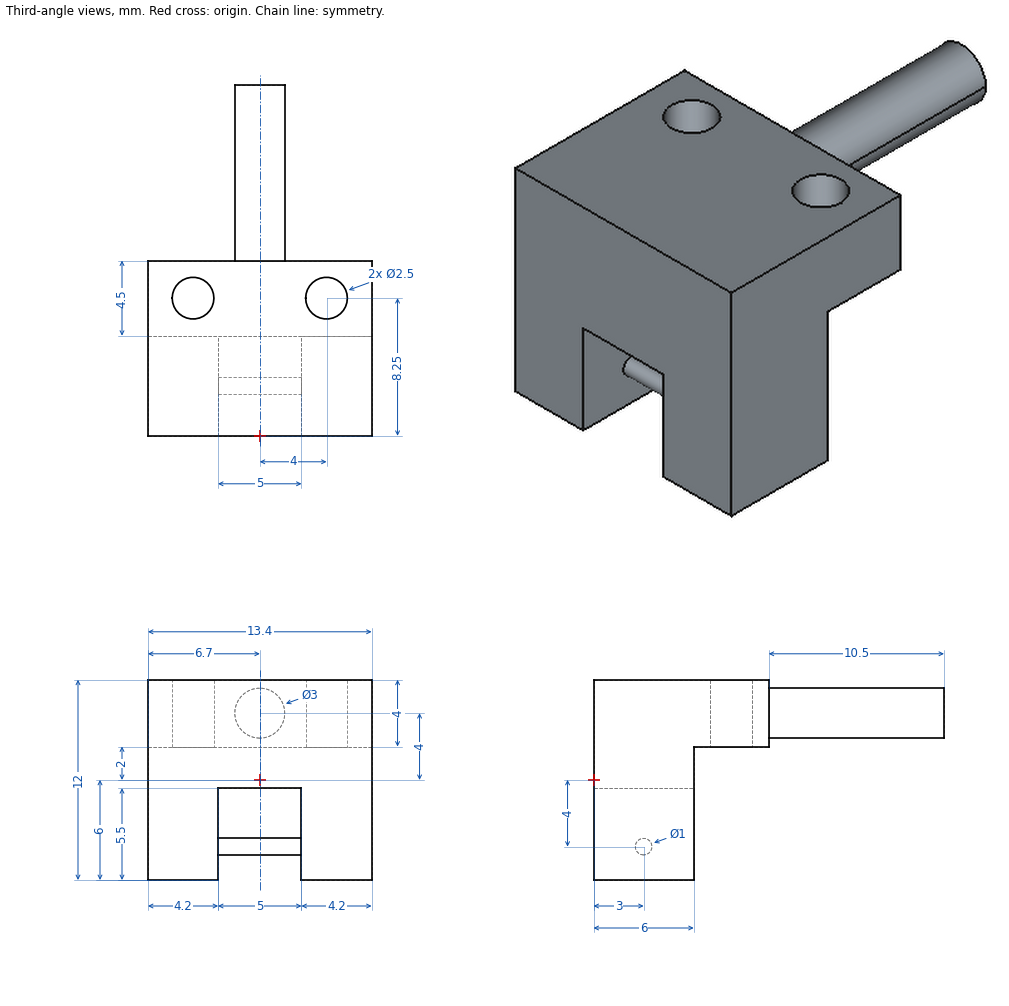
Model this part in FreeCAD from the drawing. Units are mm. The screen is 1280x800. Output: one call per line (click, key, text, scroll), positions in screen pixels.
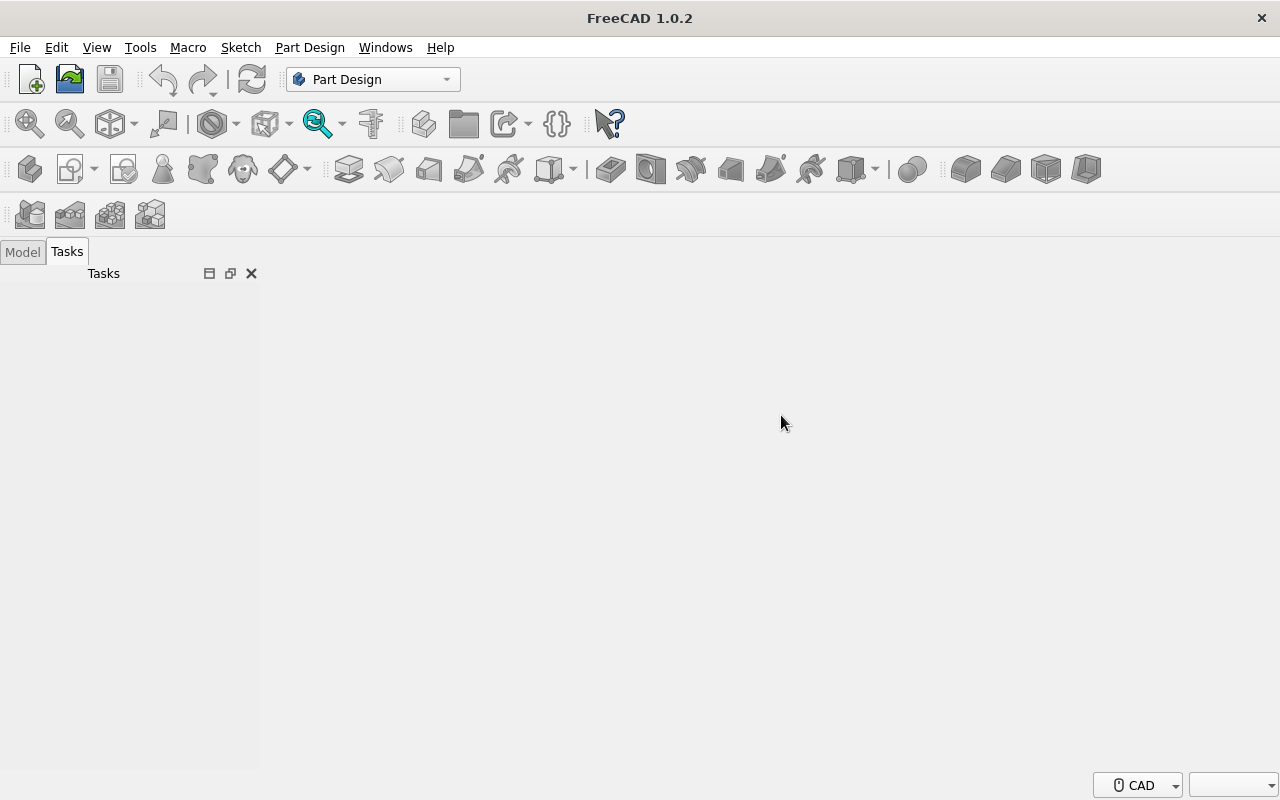
click(30, 80)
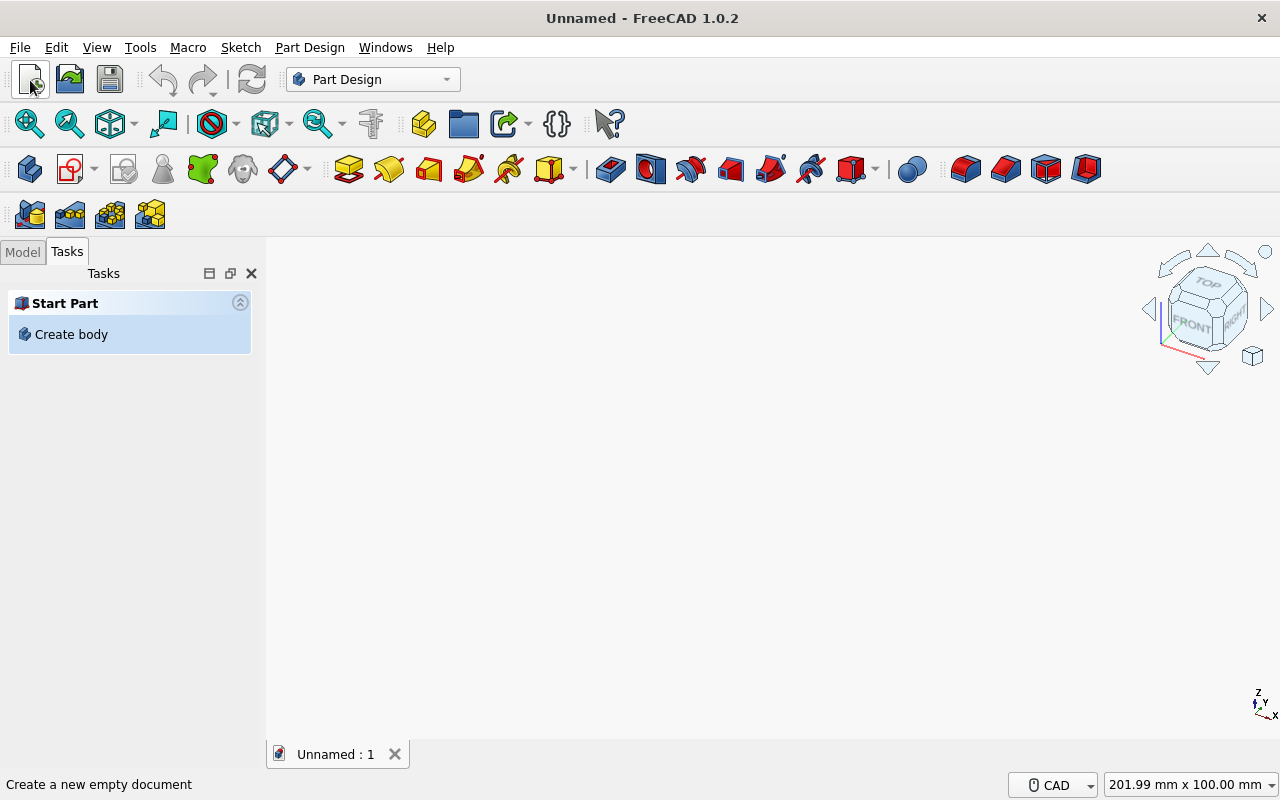
click(70, 170)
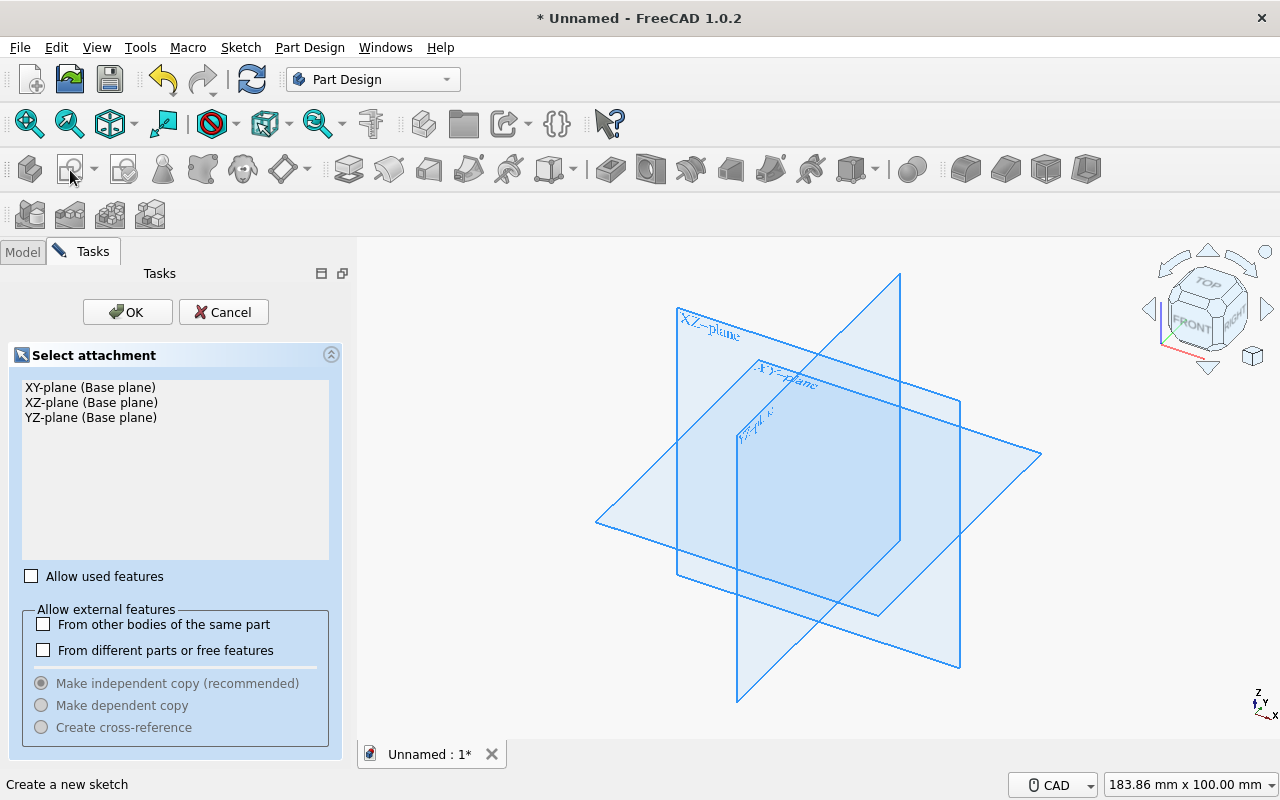
click(82, 402)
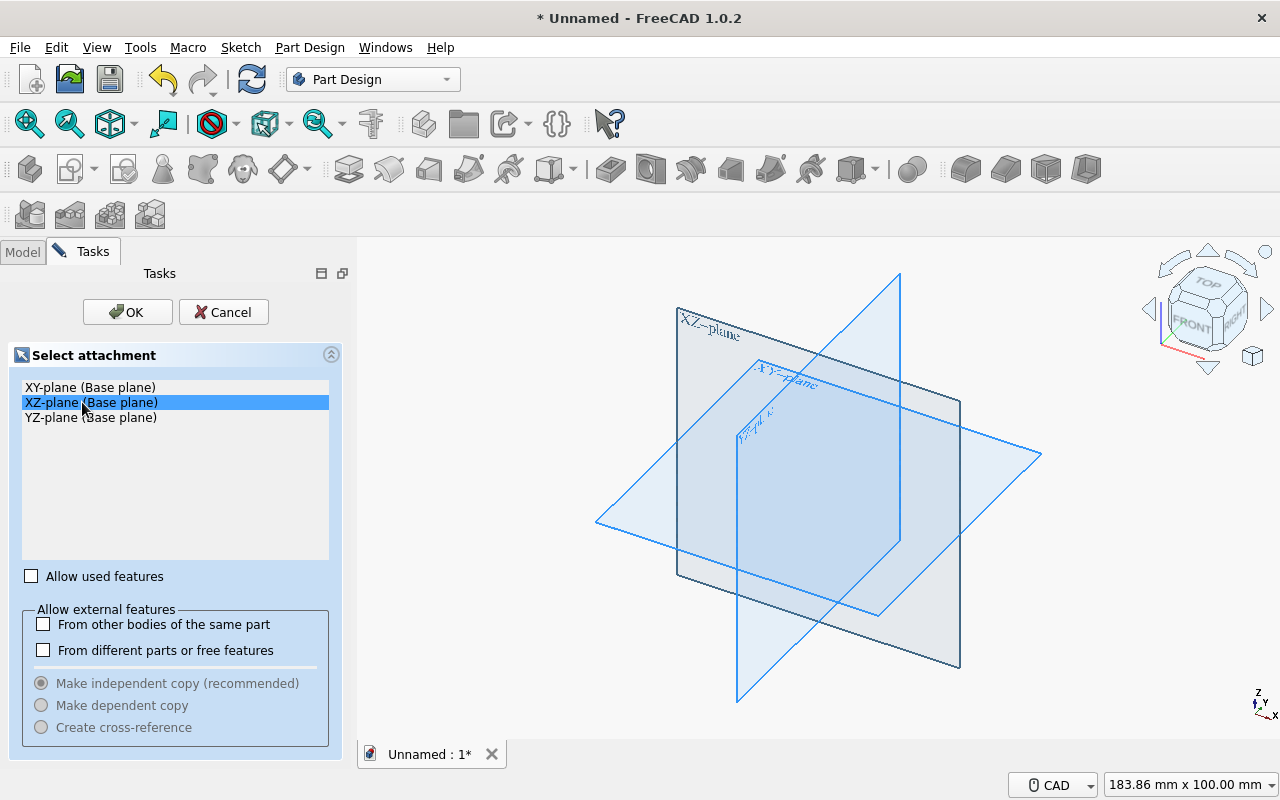
click(128, 312)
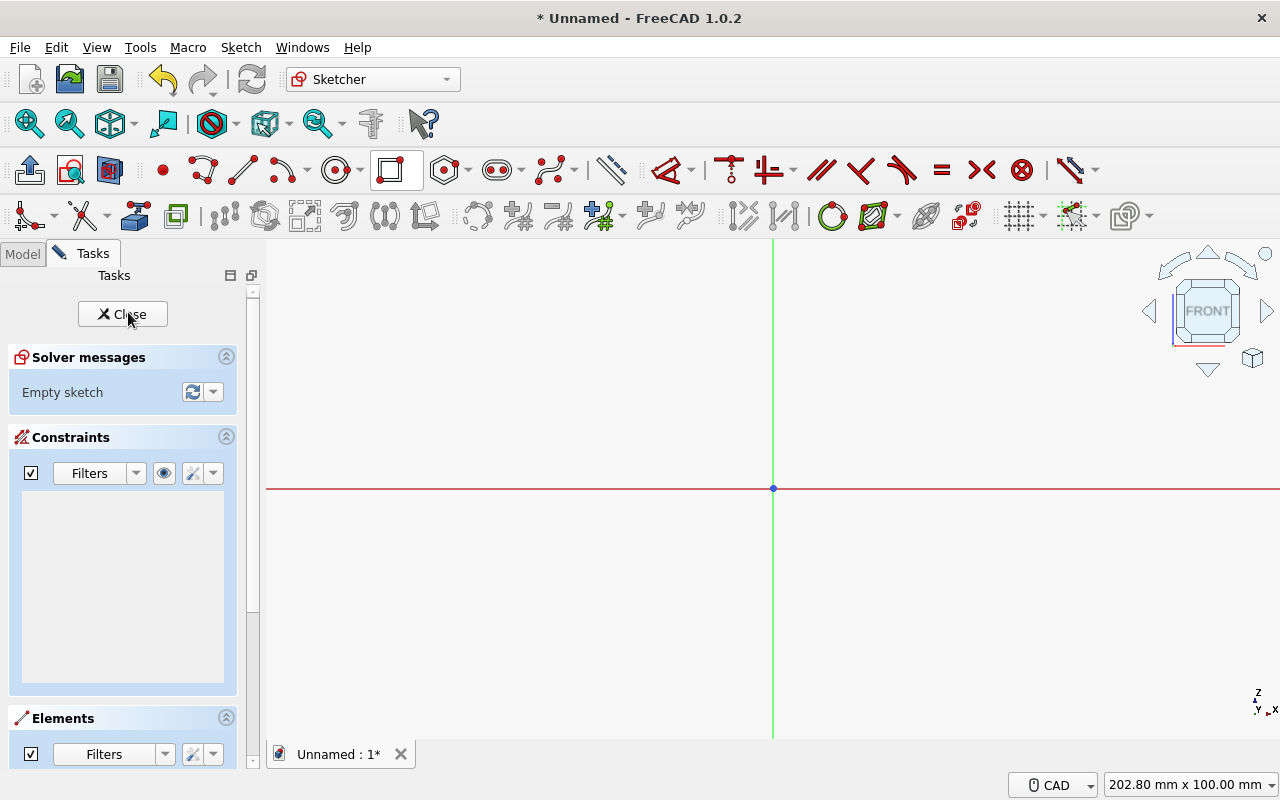
scroll(790, 489, up, 8)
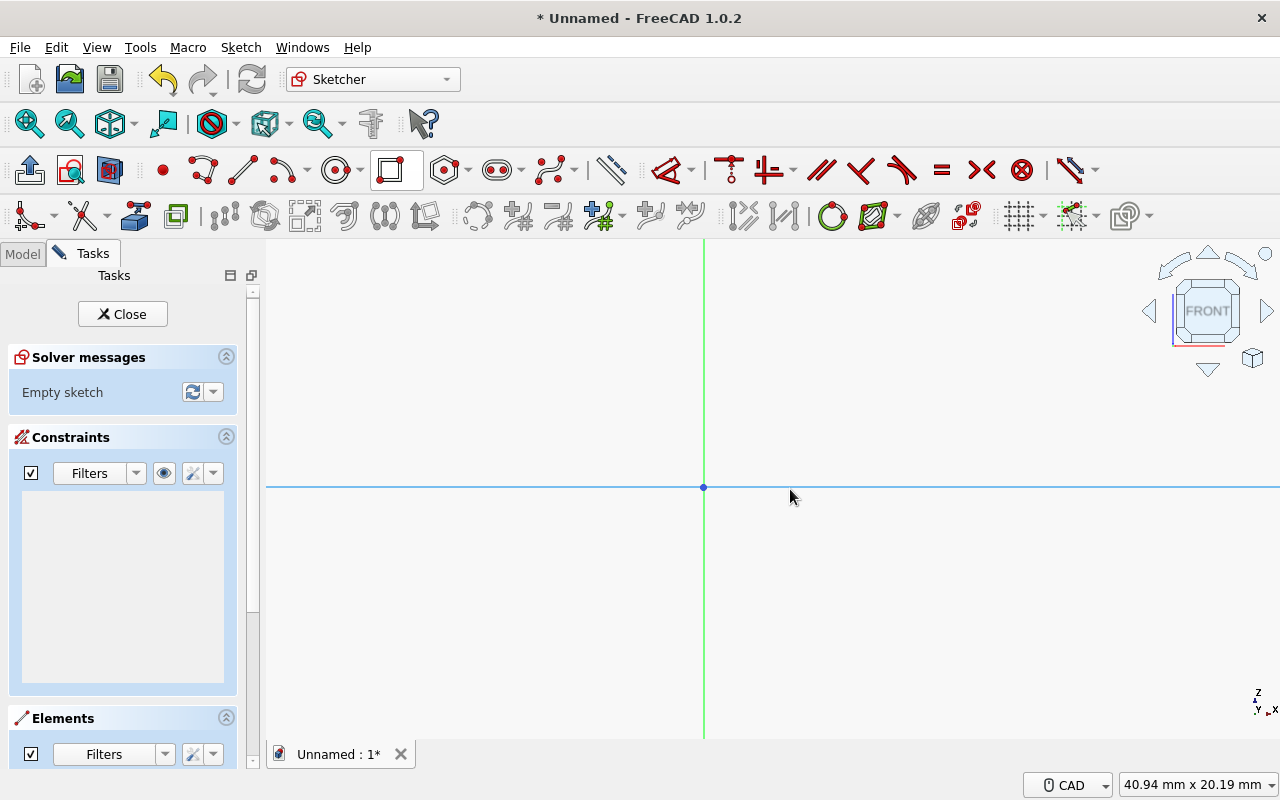
click(204, 170)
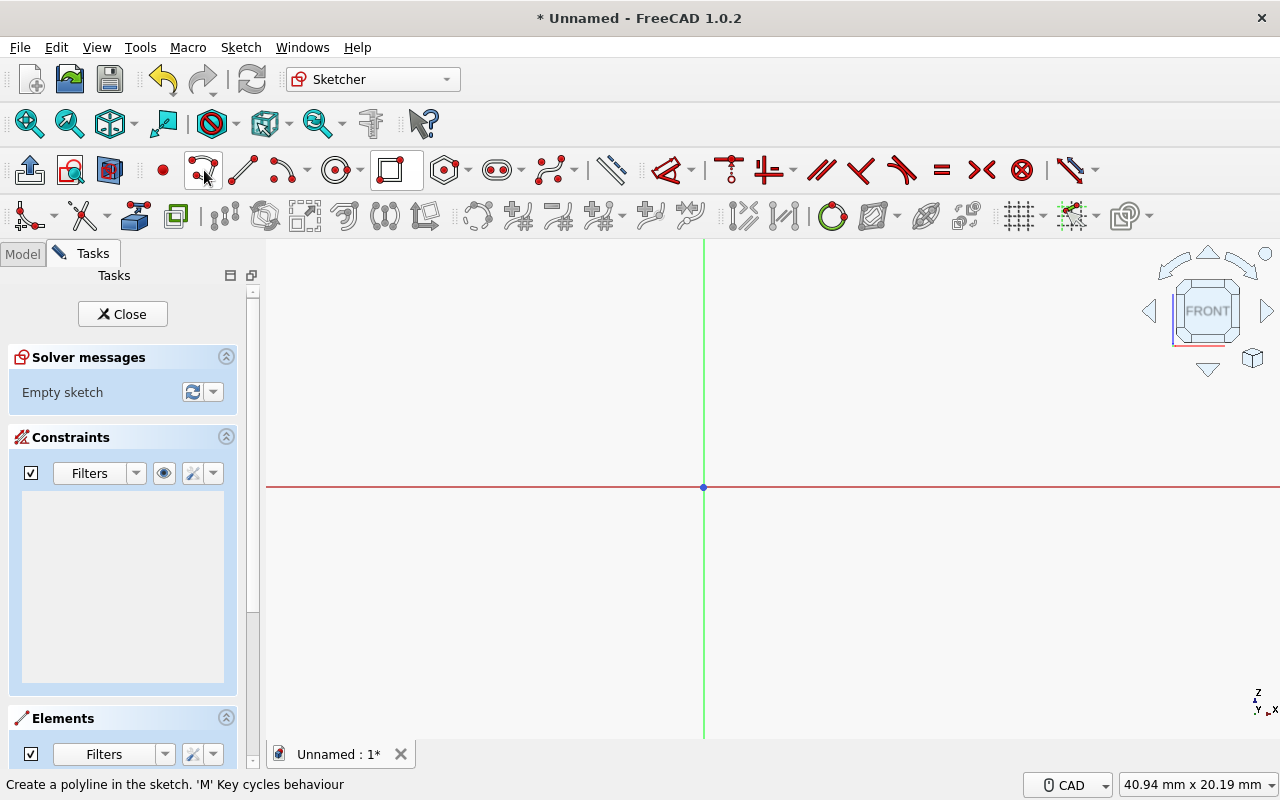
scroll(766, 499, up, 2)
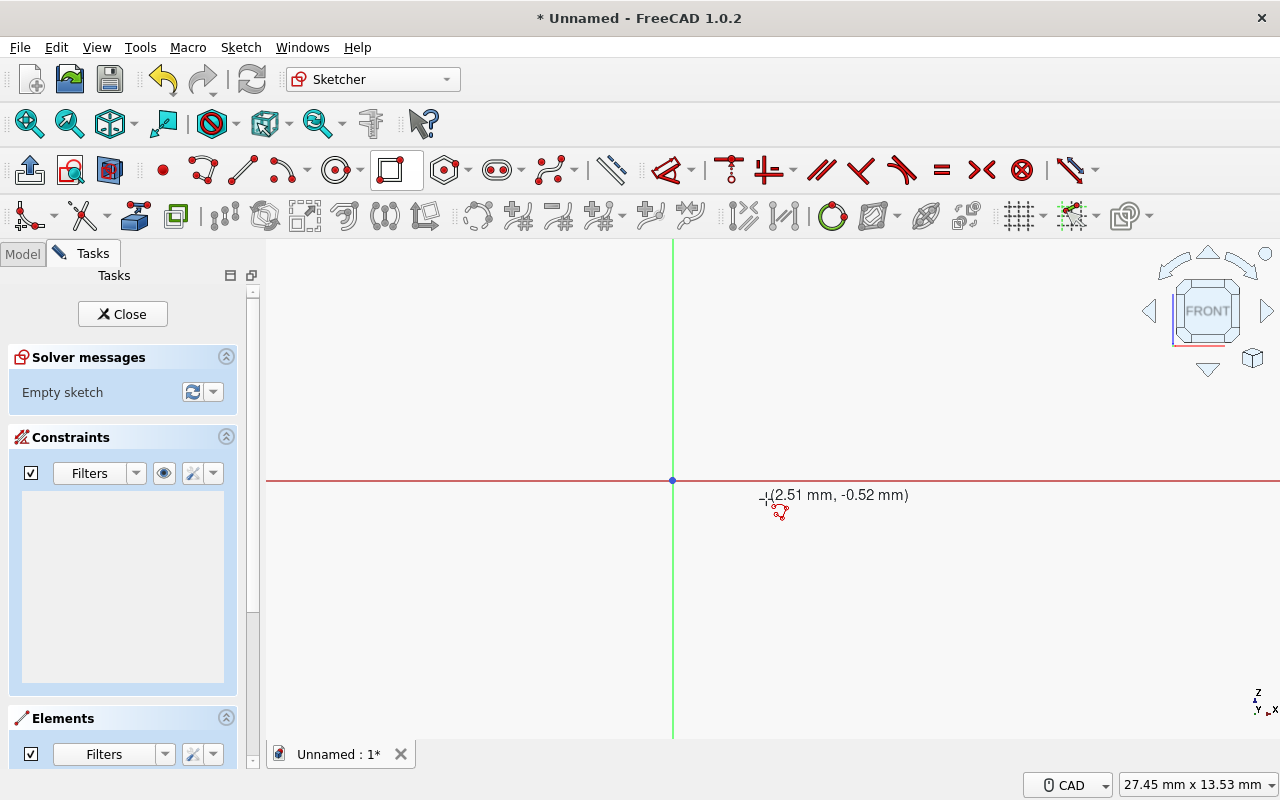
click(765, 499)
click(581, 499)
click(581, 703)
click(425, 703)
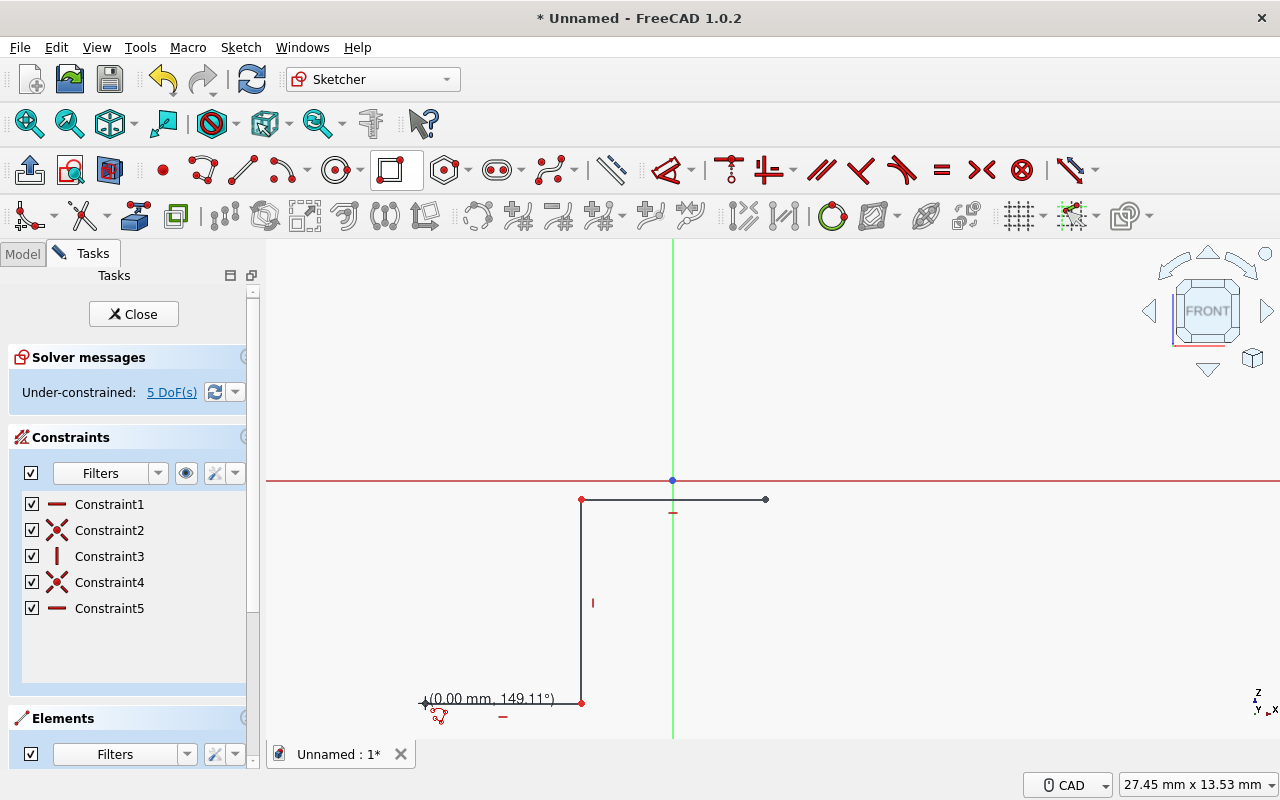
scroll(769, 506, down, 2)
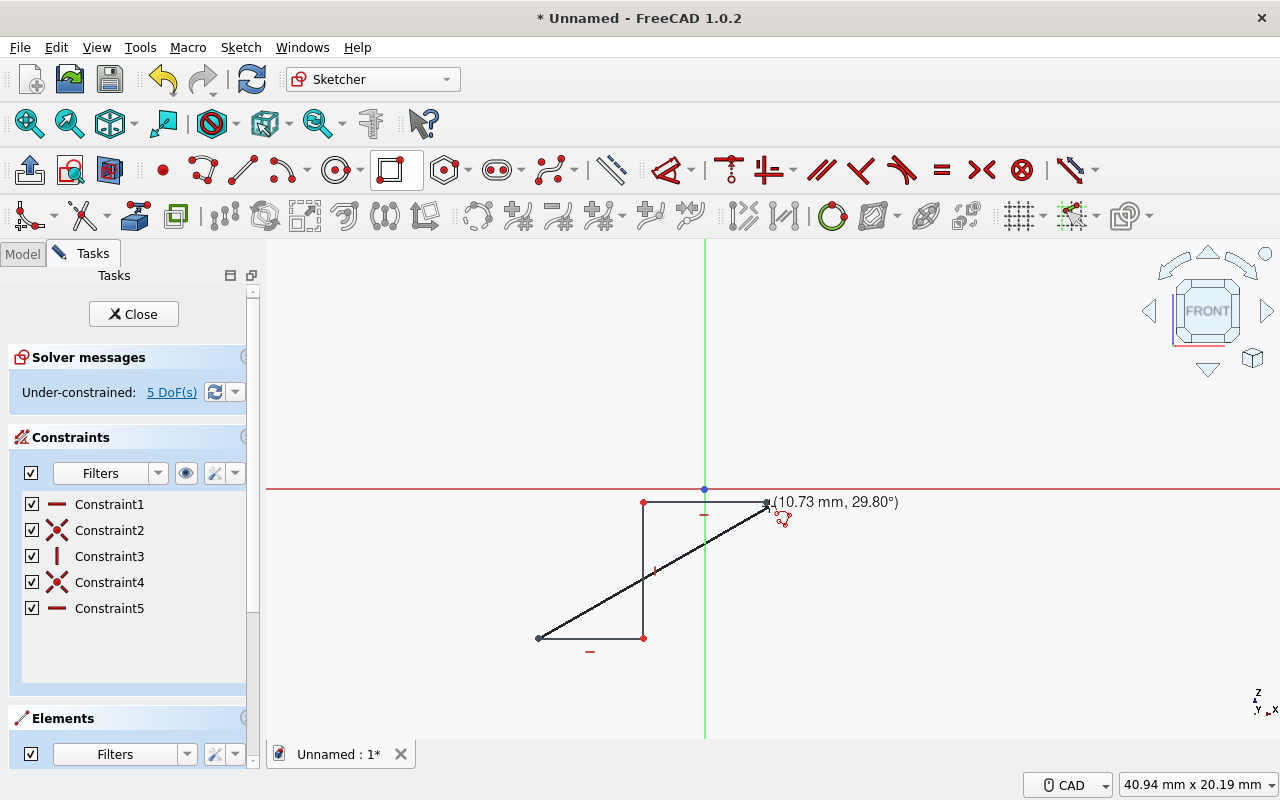
click(539, 341)
click(871, 341)
click(871, 638)
click(767, 638)